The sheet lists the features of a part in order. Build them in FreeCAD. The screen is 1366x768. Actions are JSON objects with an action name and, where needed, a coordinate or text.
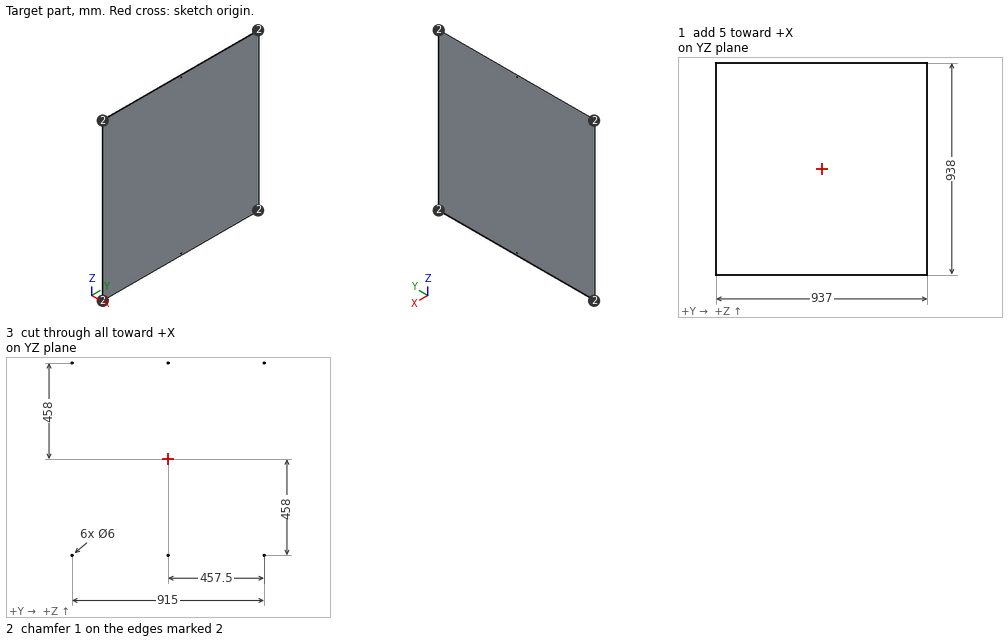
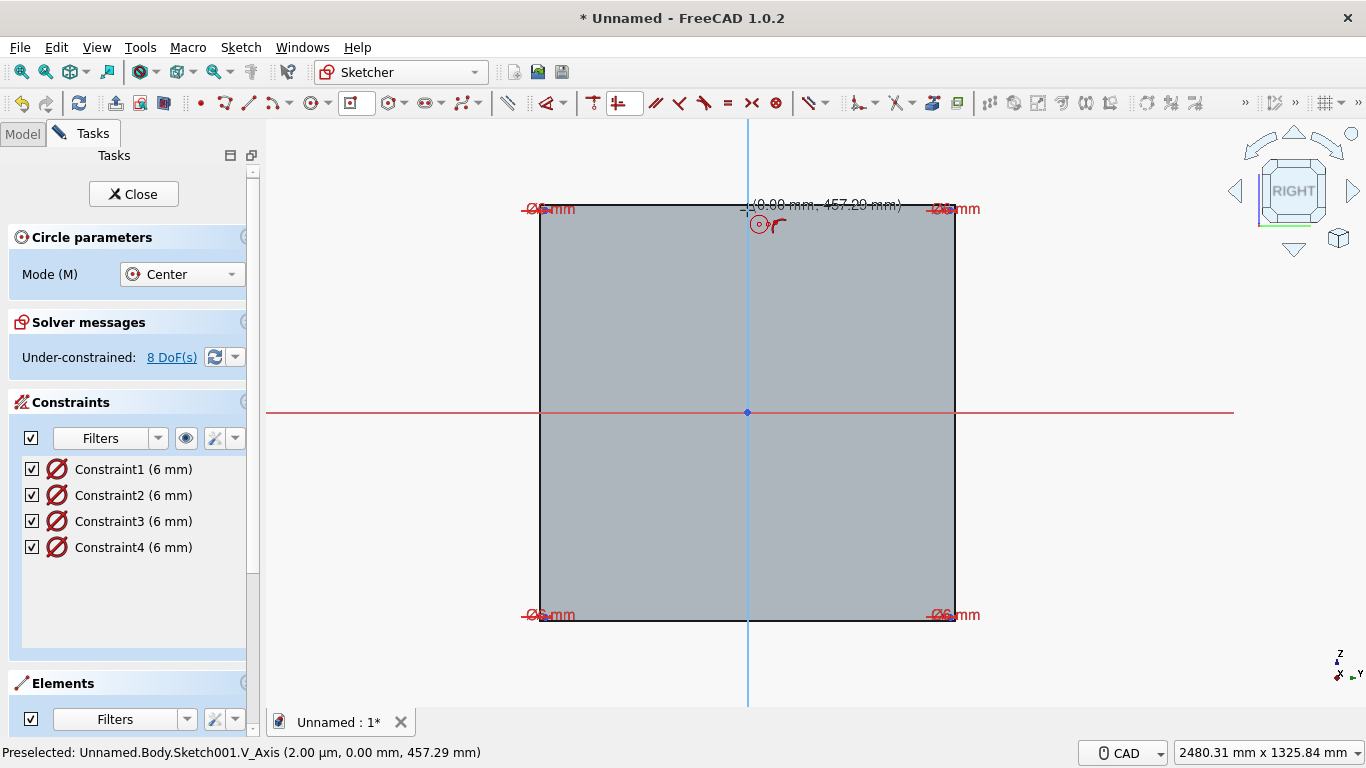
{"action": "left_click", "coordinate": [748, 210]}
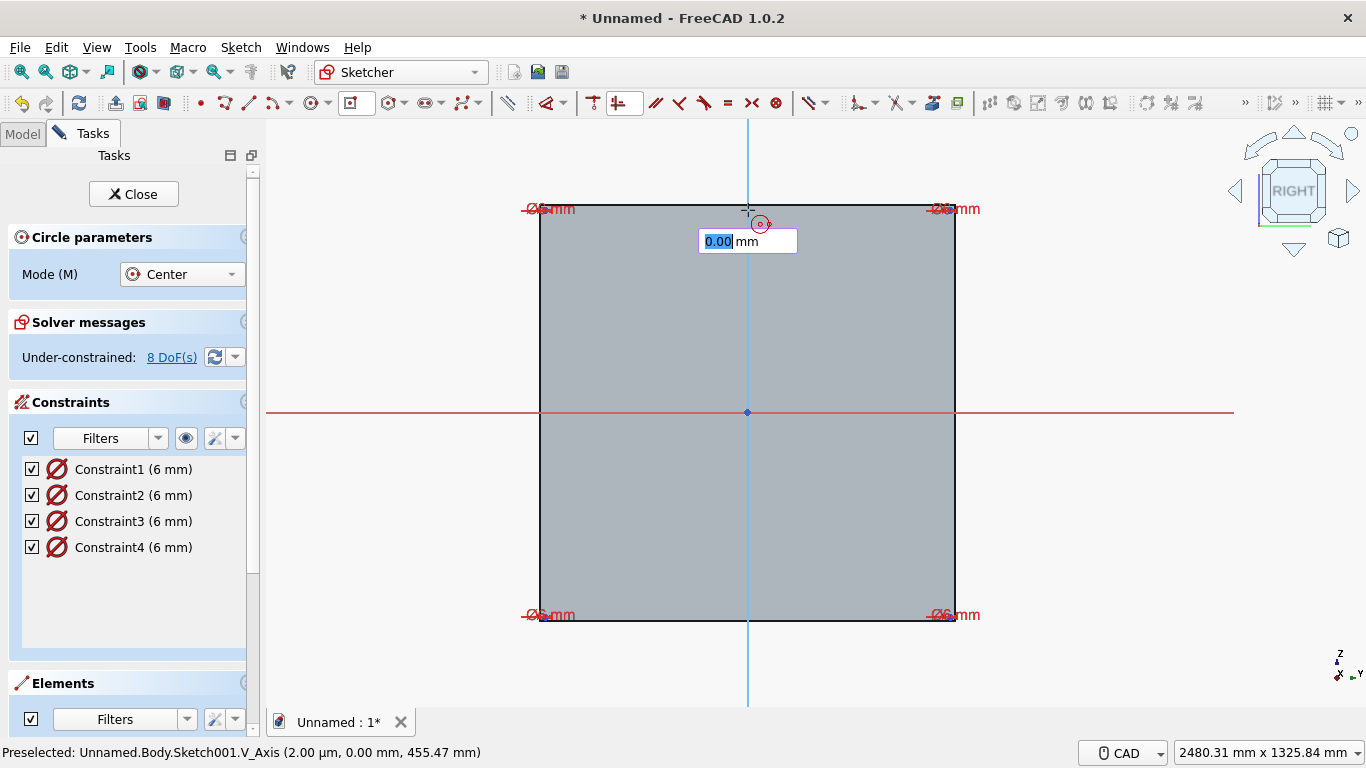
{"action": "scroll", "coordinate": [749, 209], "scroll_direction": "up", "scroll_amount": 13}
{"action": "mouse_move", "coordinate": [740, 213]}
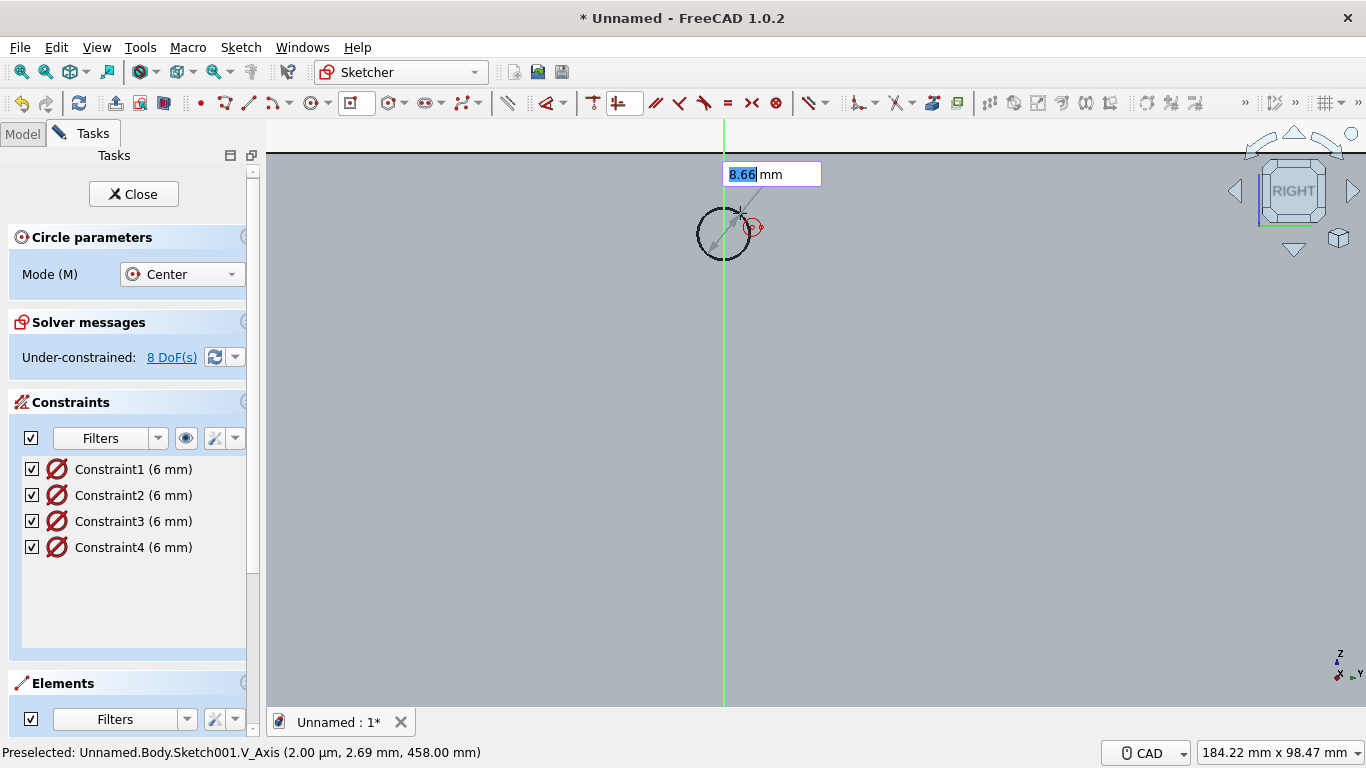
{"action": "type", "text": "6"}
{"action": "key", "text": "Return"}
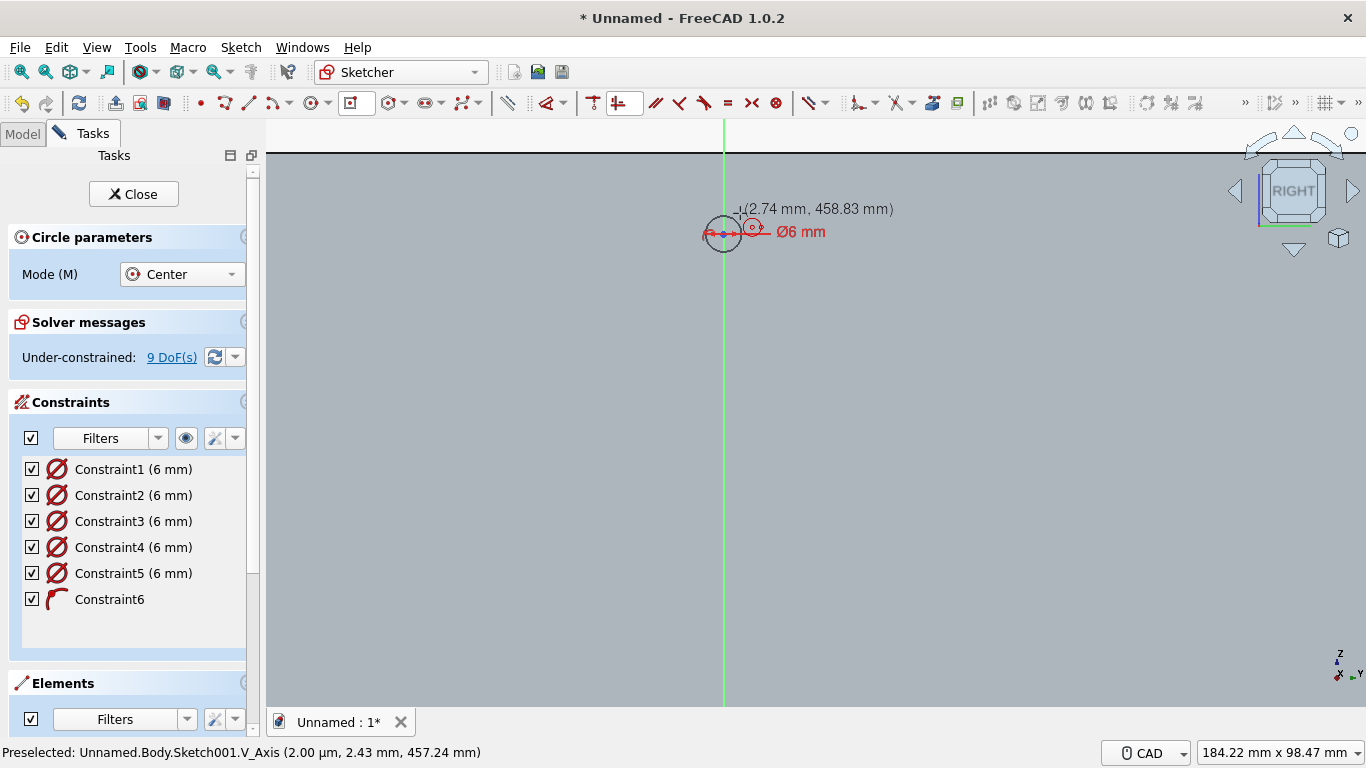
{"action": "scroll", "coordinate": [749, 209], "scroll_direction": "down", "scroll_amount": 13}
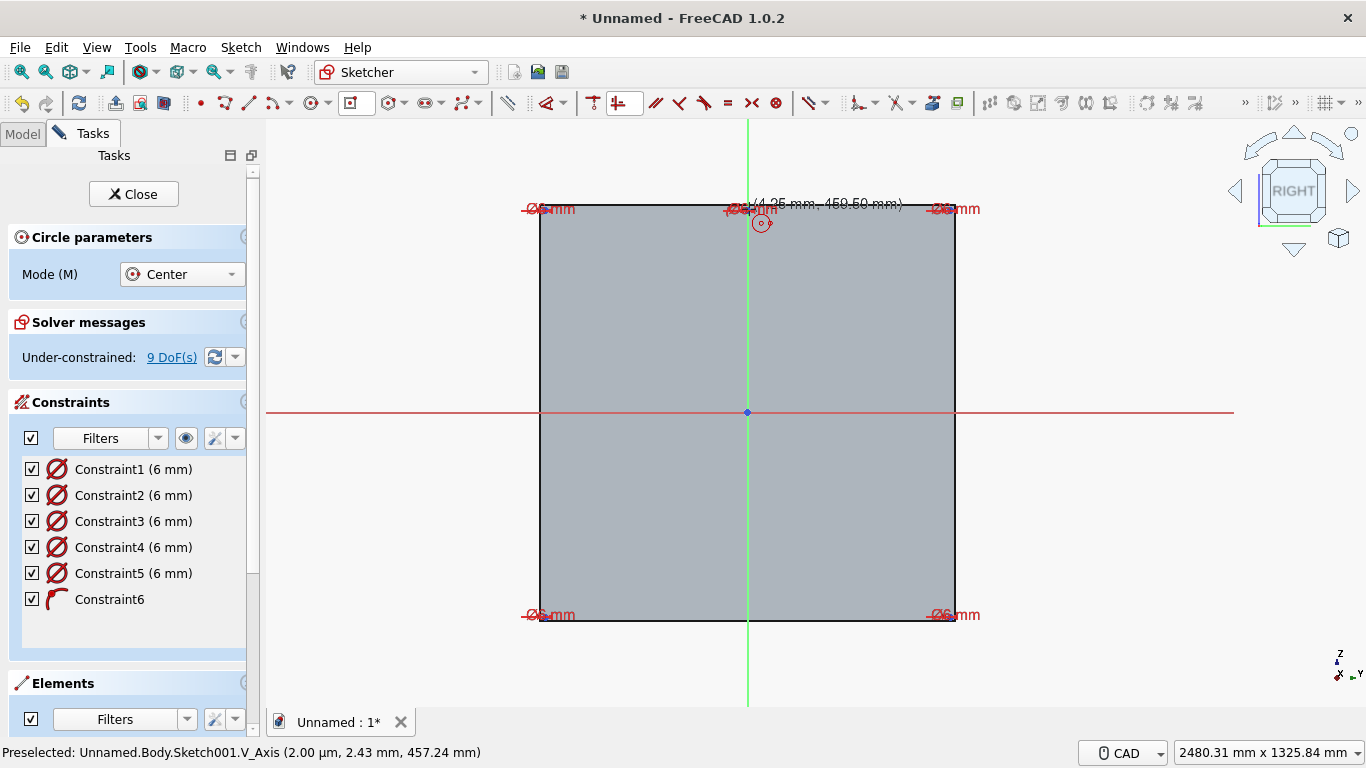
{"action": "scroll", "coordinate": [748, 616], "scroll_direction": "up", "scroll_amount": 15}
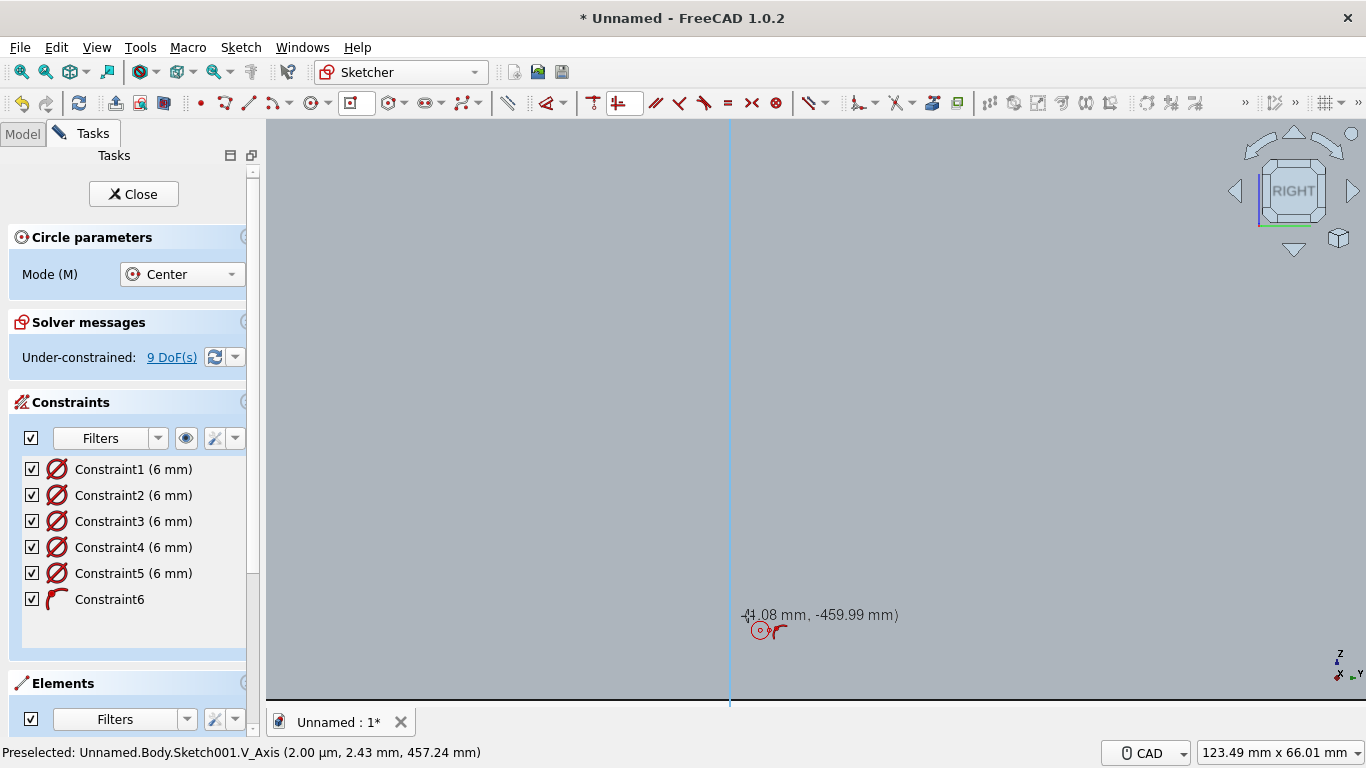
{"action": "scroll", "coordinate": [748, 617], "scroll_direction": "down", "scroll_amount": 15}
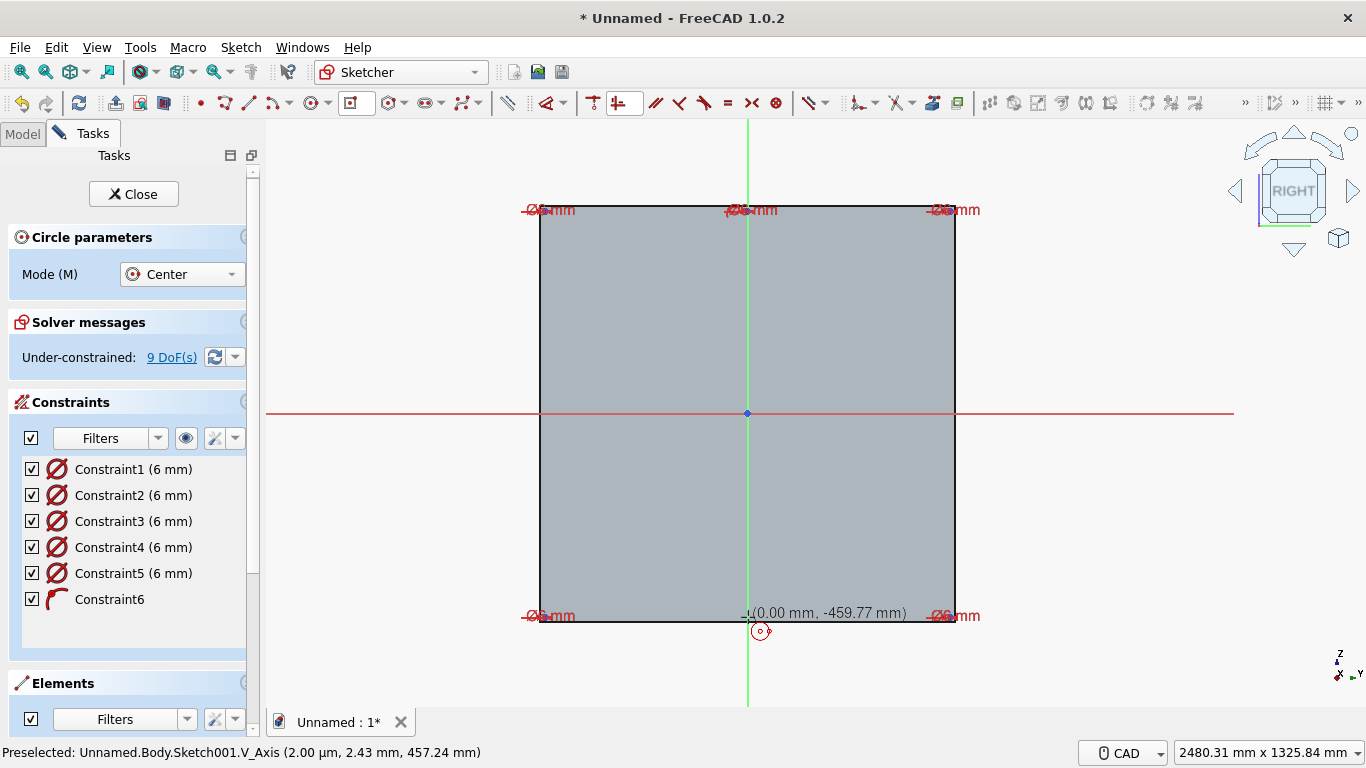
{"action": "left_click", "coordinate": [748, 617]}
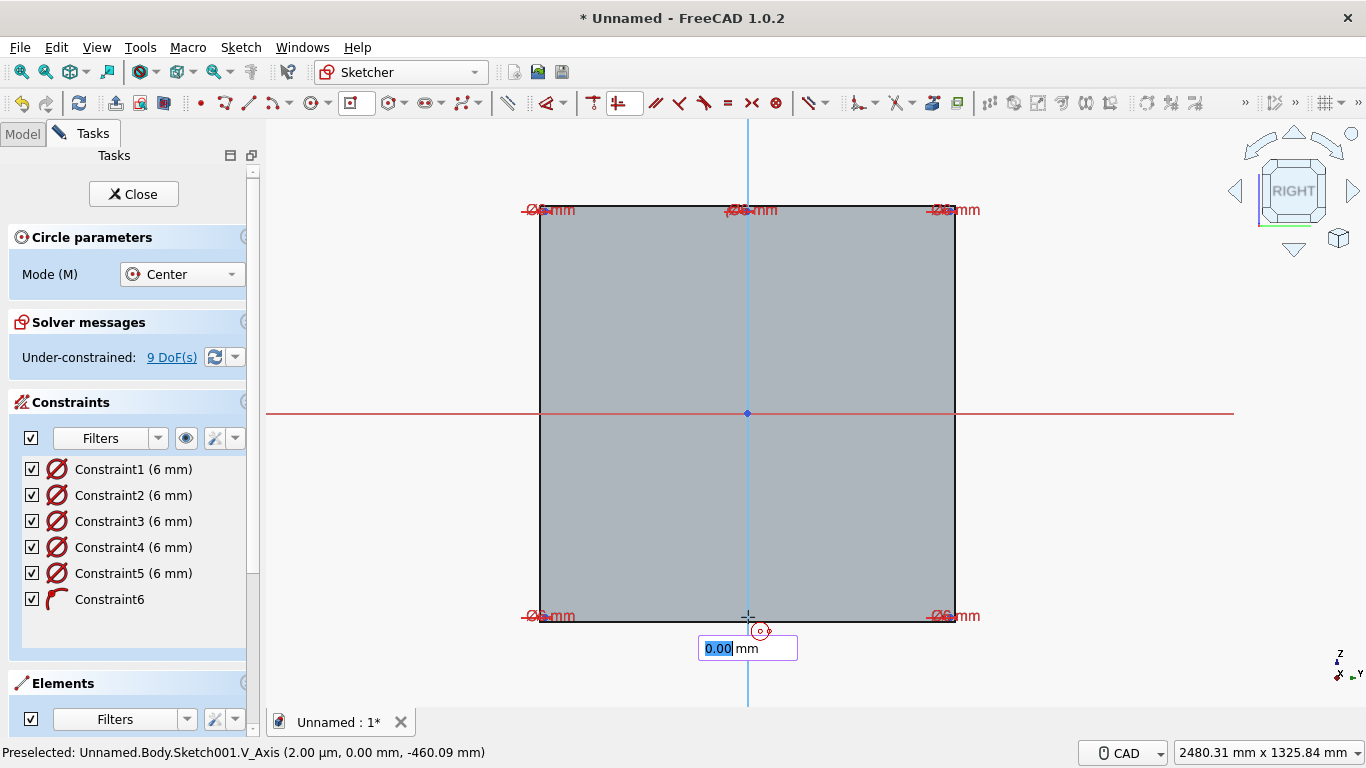
{"action": "scroll", "coordinate": [749, 617], "scroll_direction": "up", "scroll_amount": 13}
{"action": "mouse_move", "coordinate": [740, 601]}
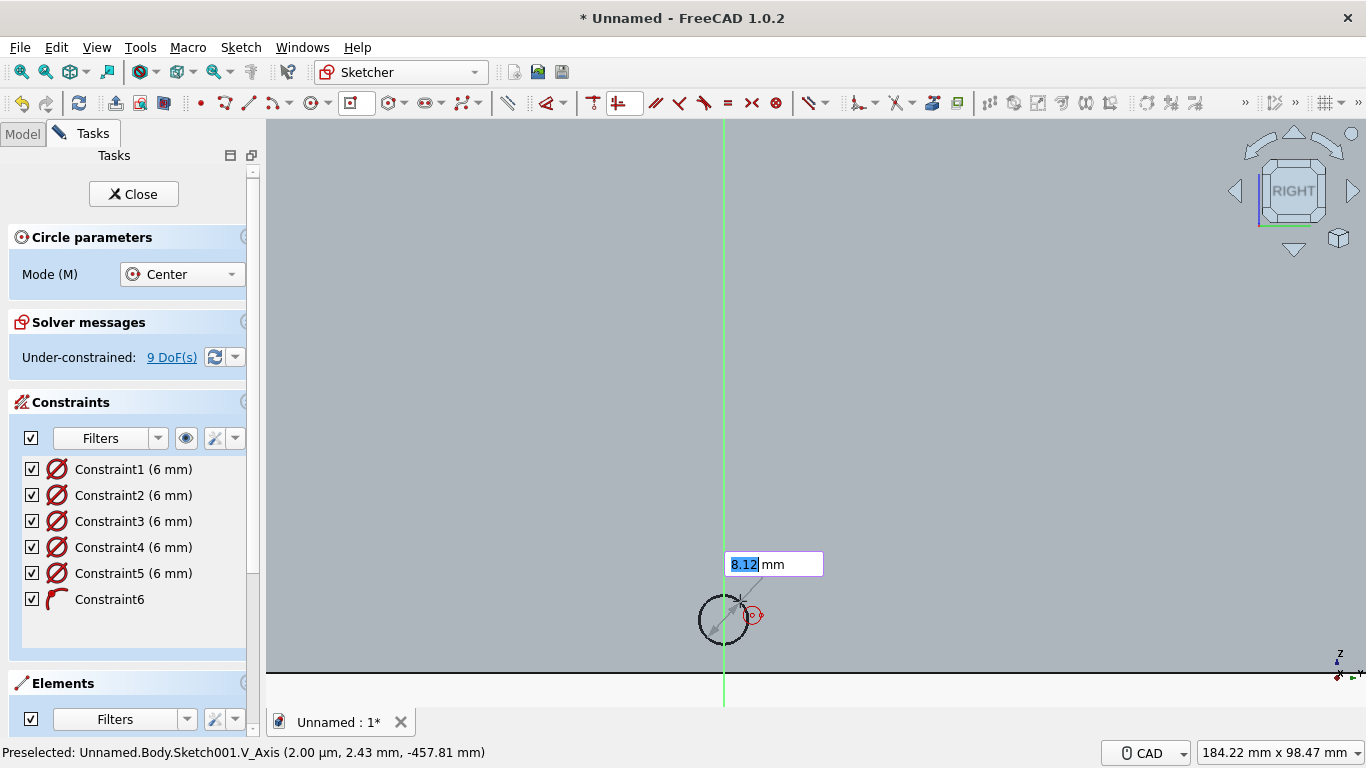
{"action": "type", "text": "6"}
{"action": "key", "text": "Return"}
{"action": "key", "text": "Escape"}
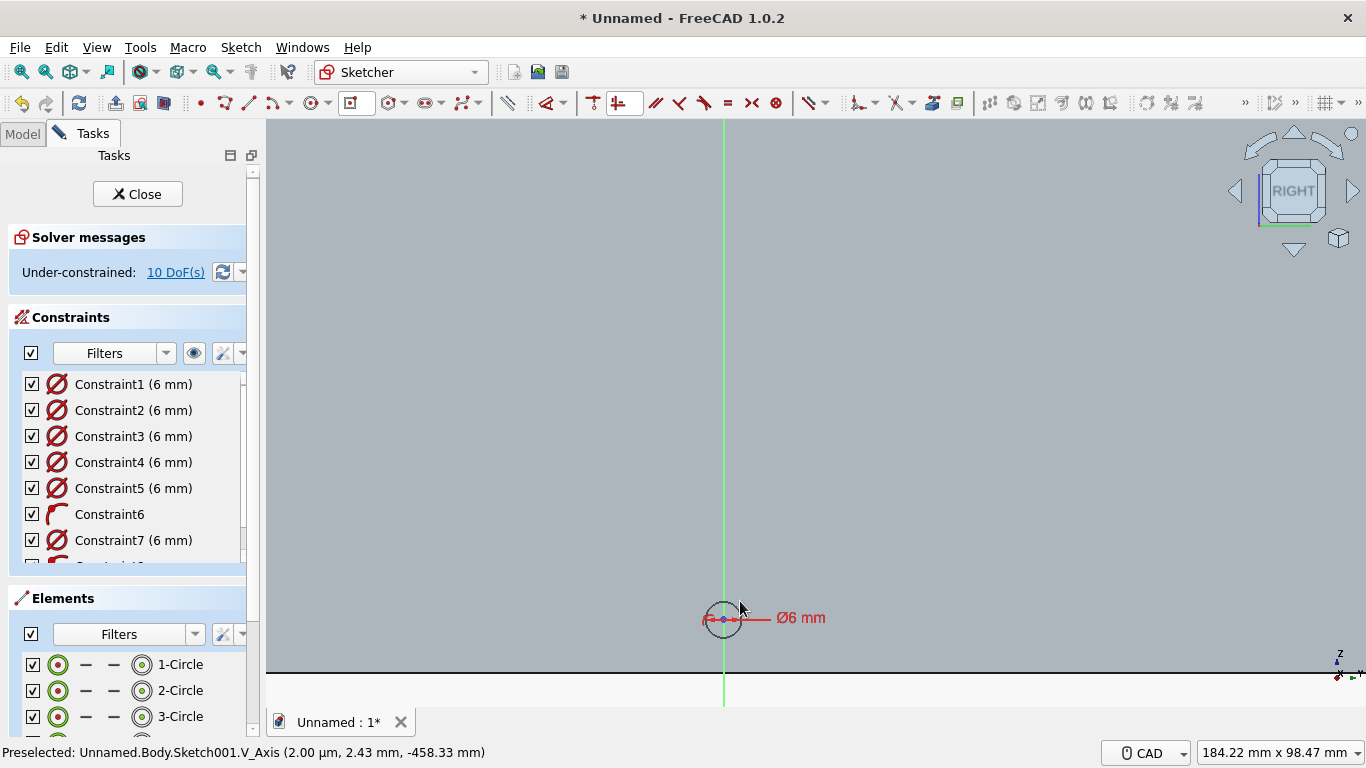
{"action": "scroll", "coordinate": [749, 617], "scroll_direction": "down", "scroll_amount": 13}